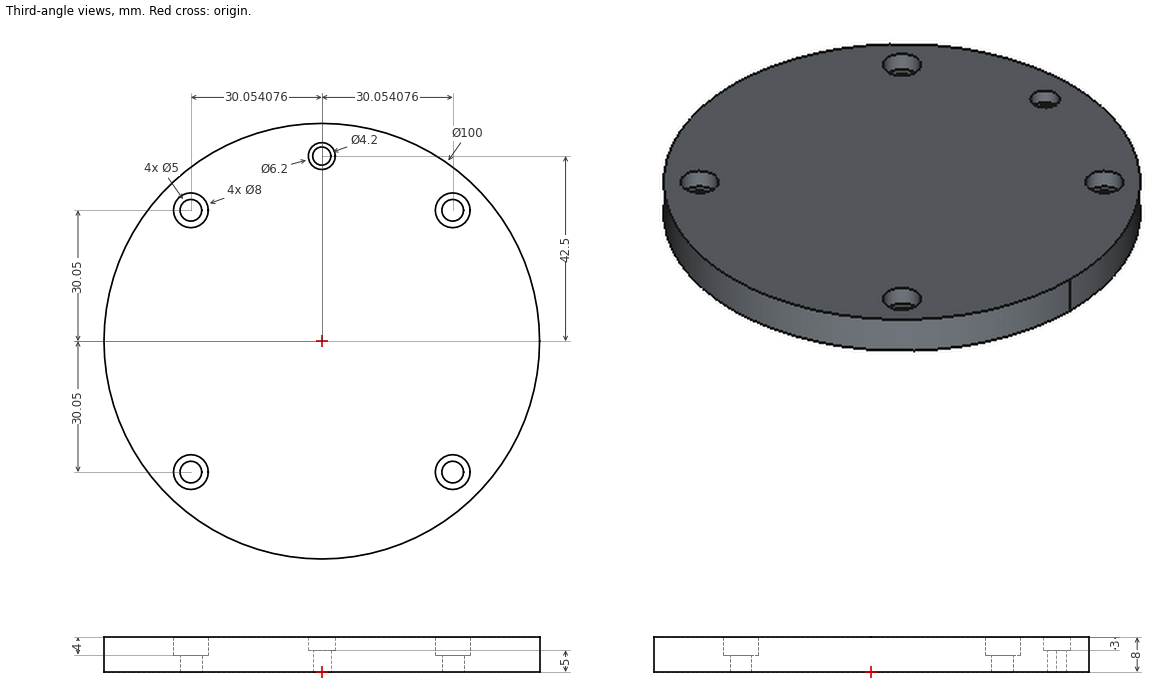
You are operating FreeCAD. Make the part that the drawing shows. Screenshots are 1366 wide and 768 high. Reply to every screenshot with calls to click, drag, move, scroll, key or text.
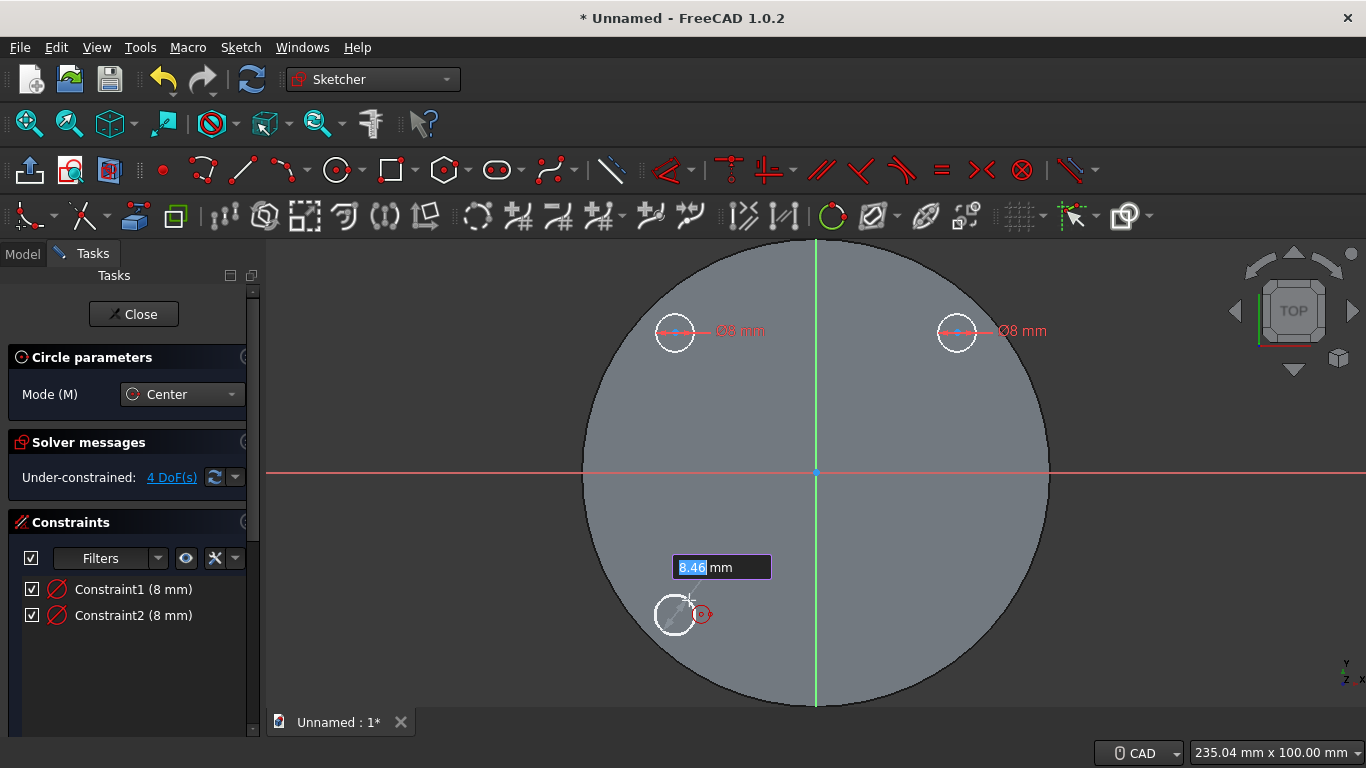
text(8)
key(Return)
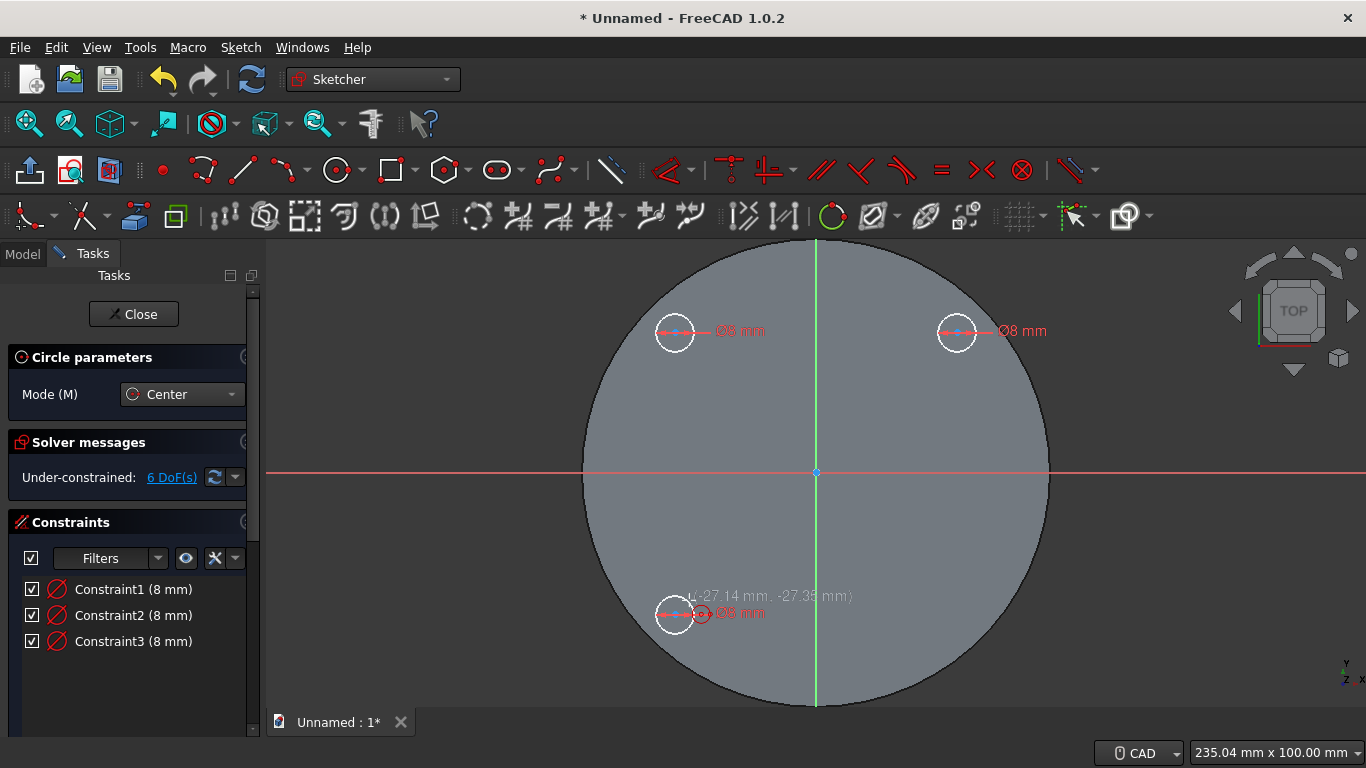
click(957, 614)
move(970, 600)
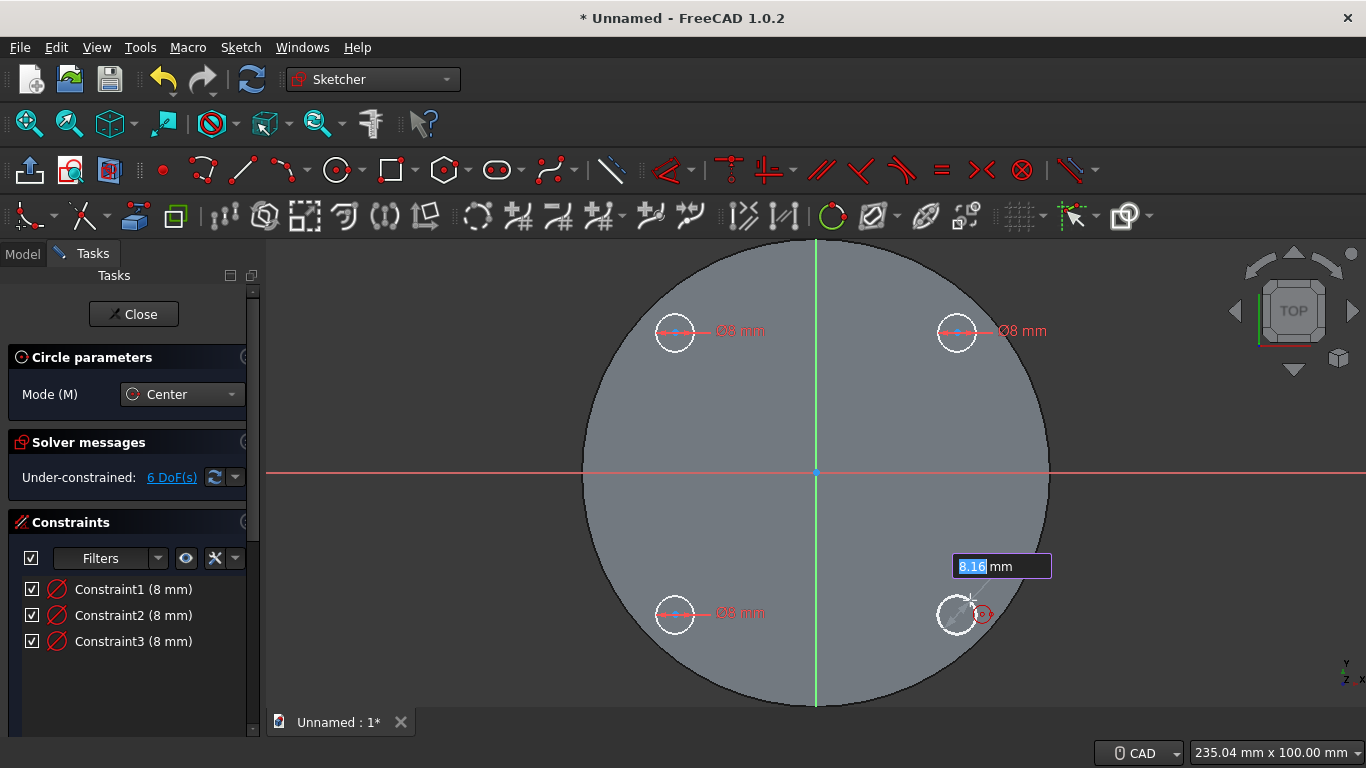
text(8)
key(Return)
key(Escape)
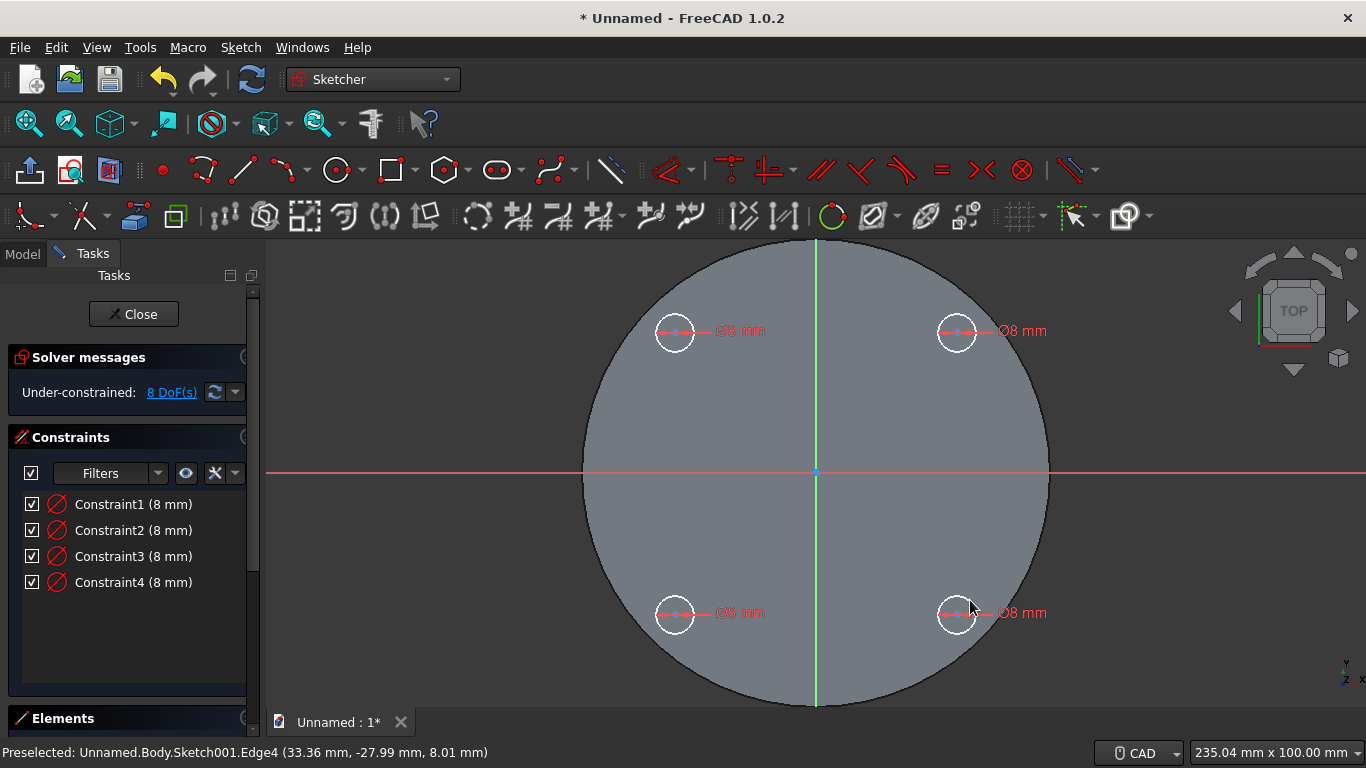
click(675, 333)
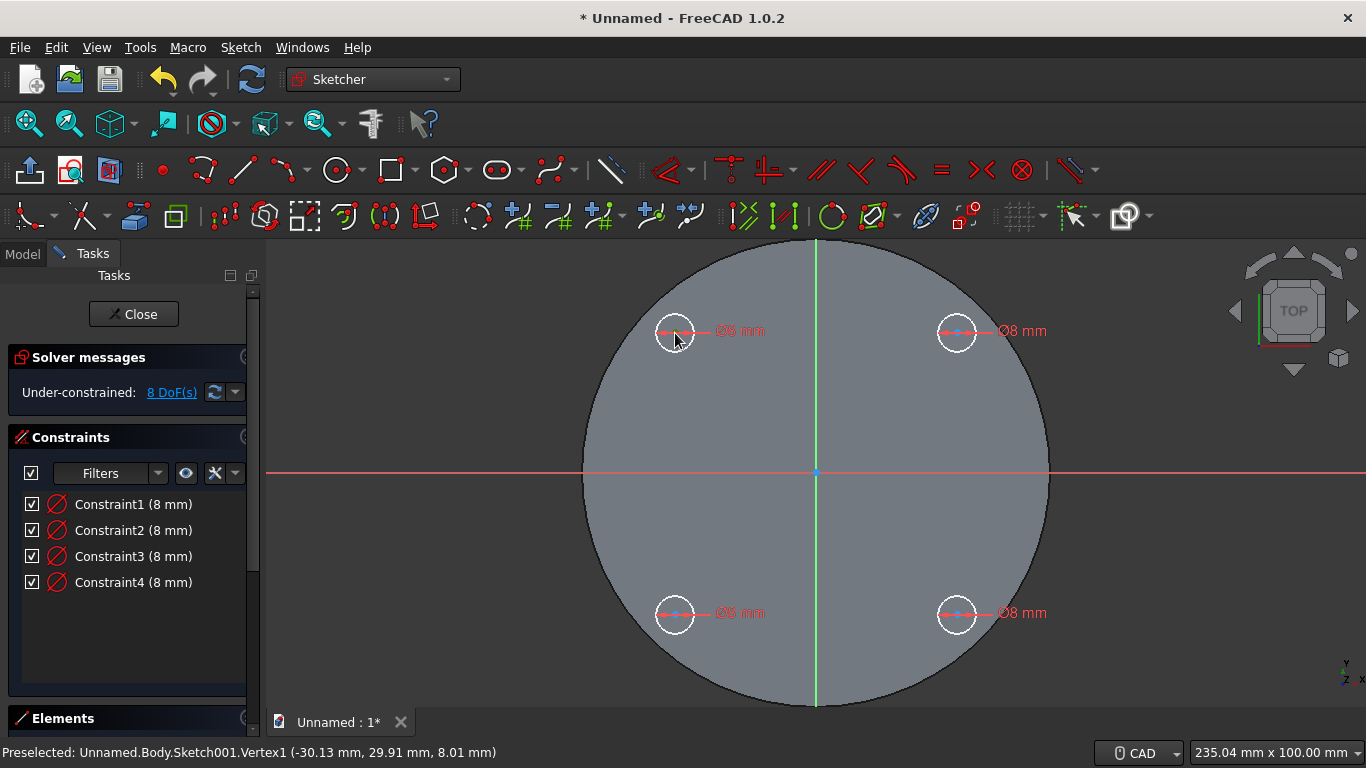
click(957, 333)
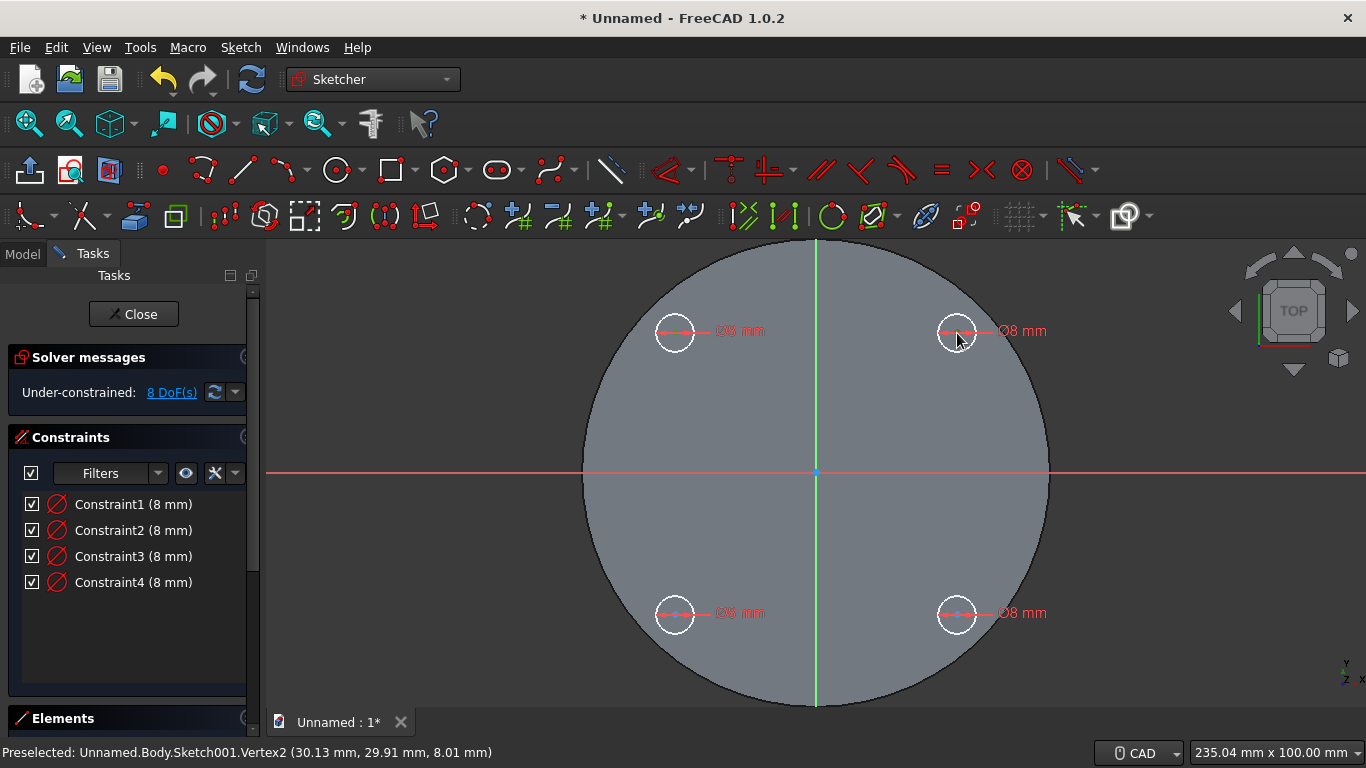
key(h)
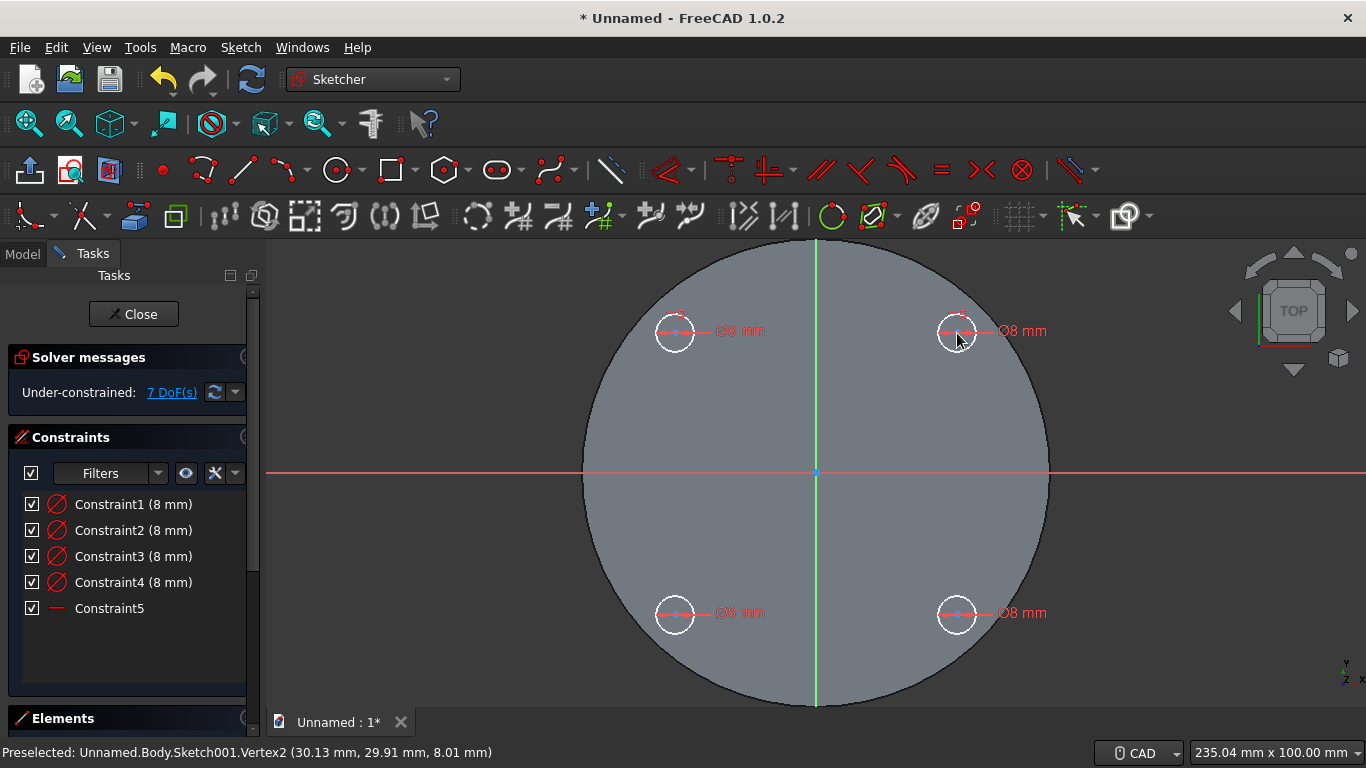
click(675, 333)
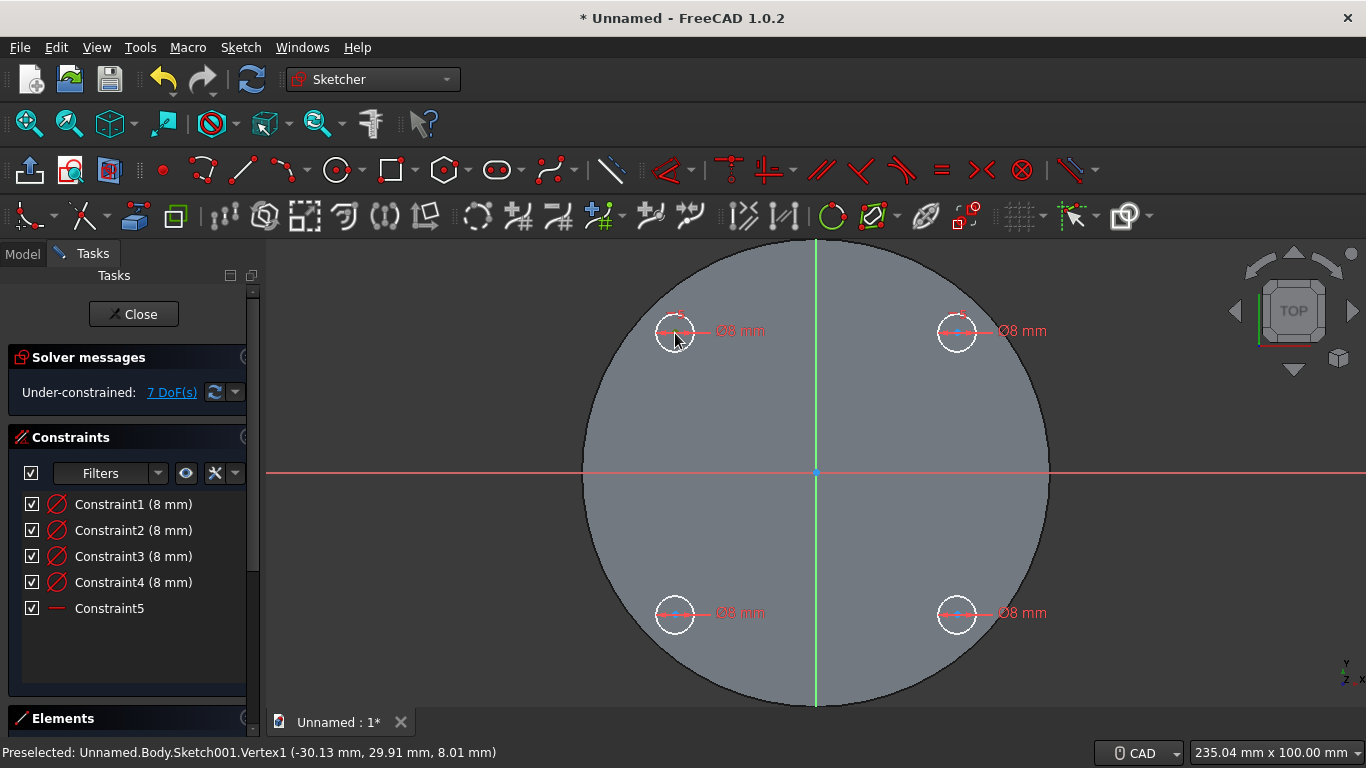
click(675, 615)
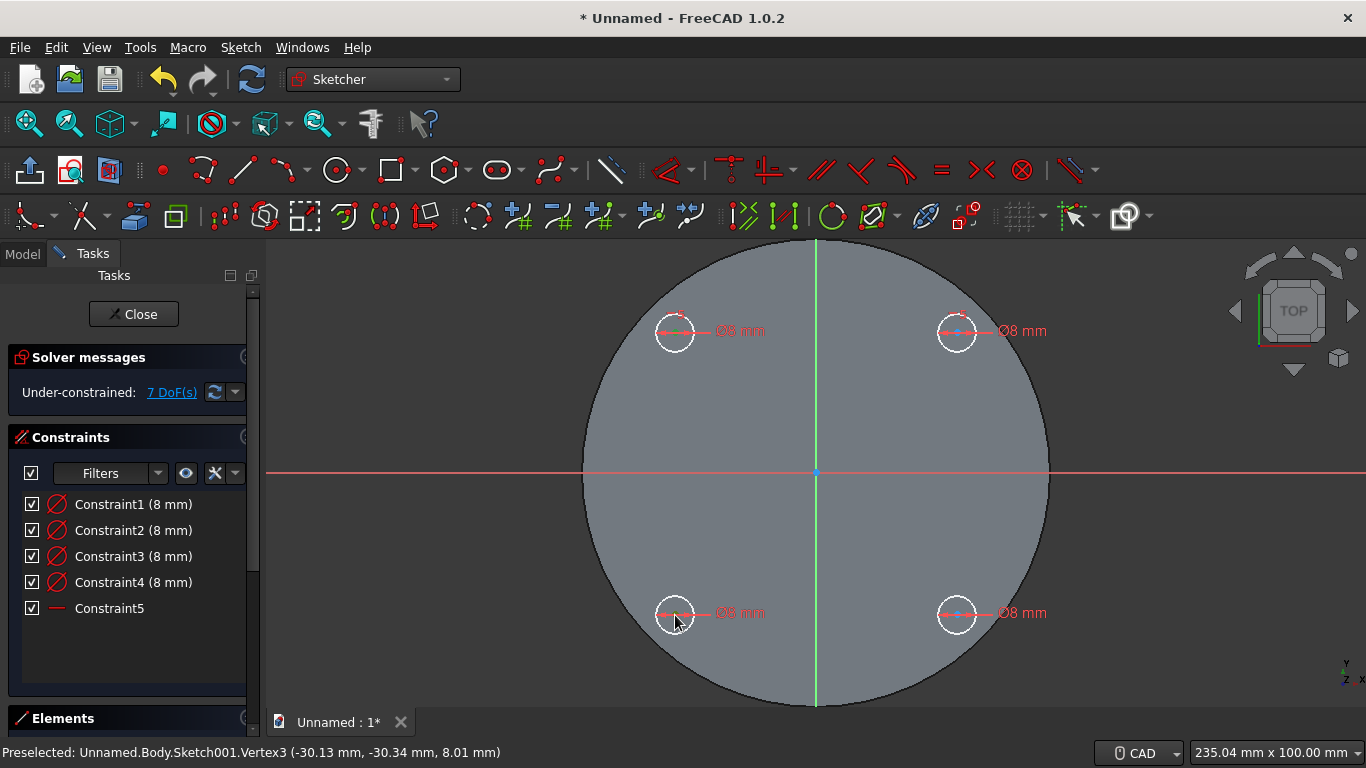
click(796, 170)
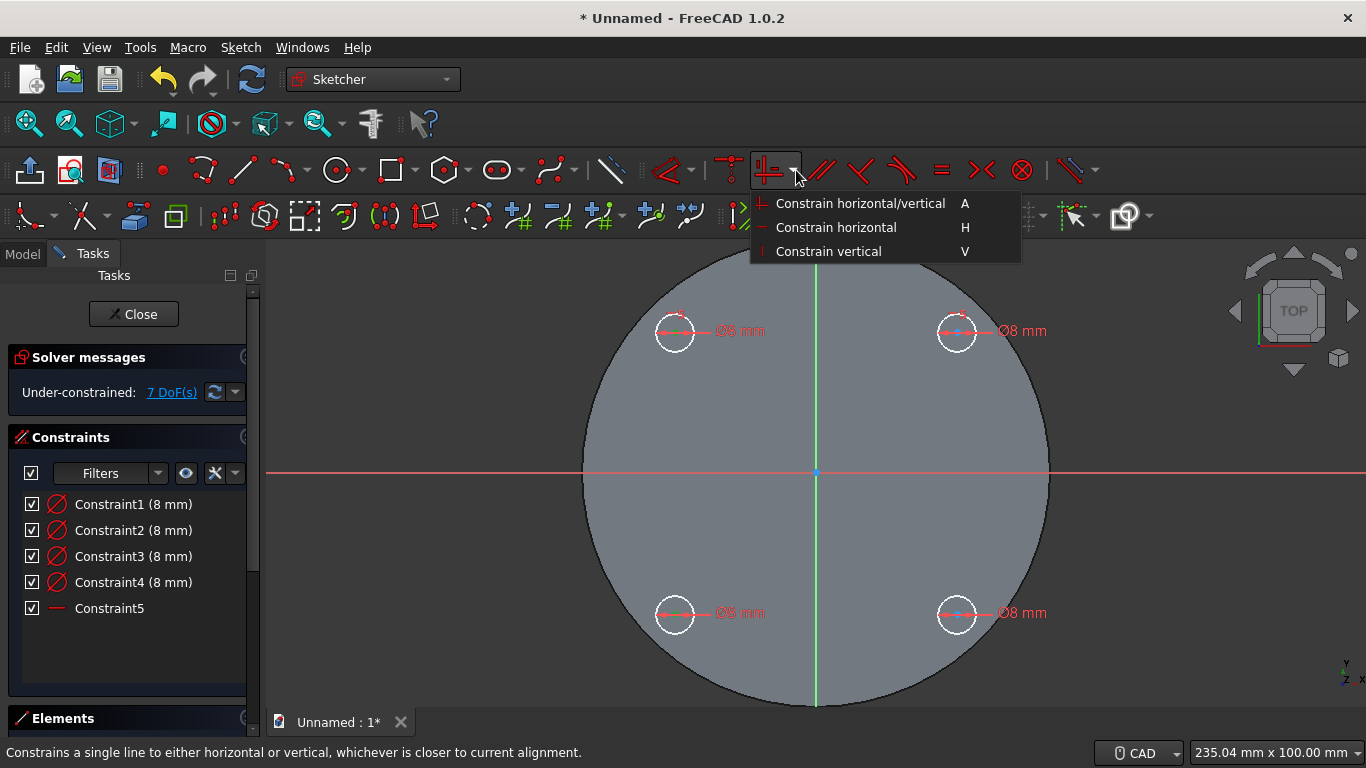
click(886, 251)